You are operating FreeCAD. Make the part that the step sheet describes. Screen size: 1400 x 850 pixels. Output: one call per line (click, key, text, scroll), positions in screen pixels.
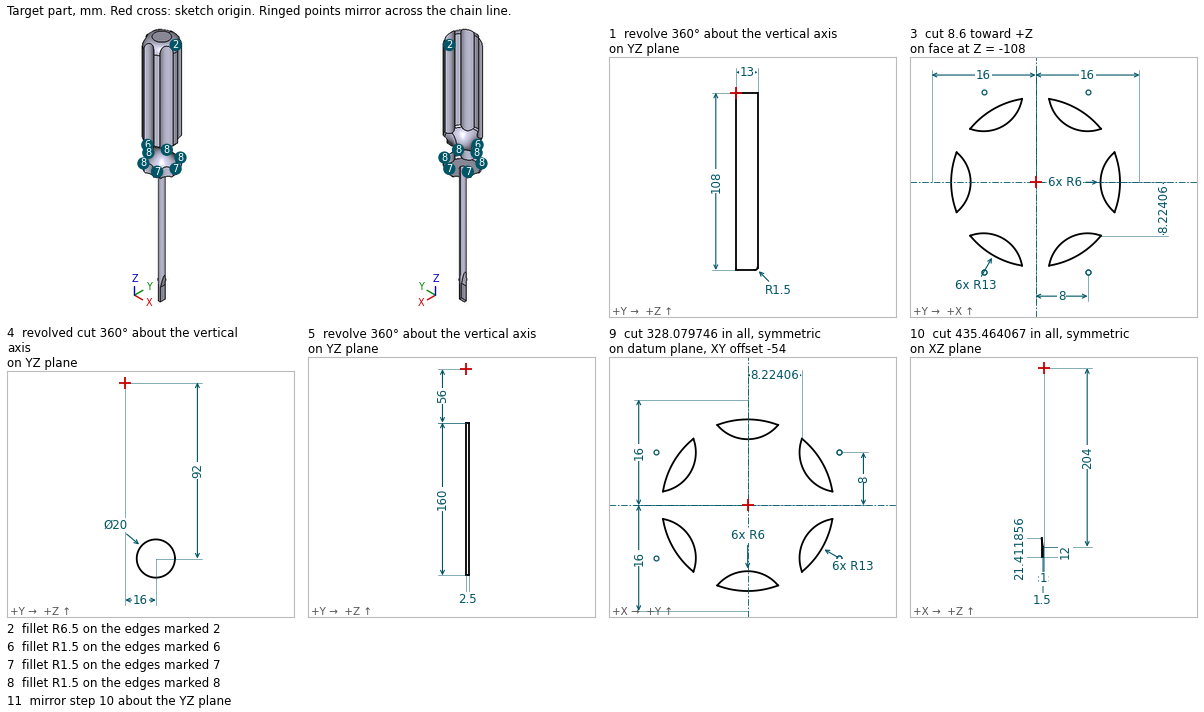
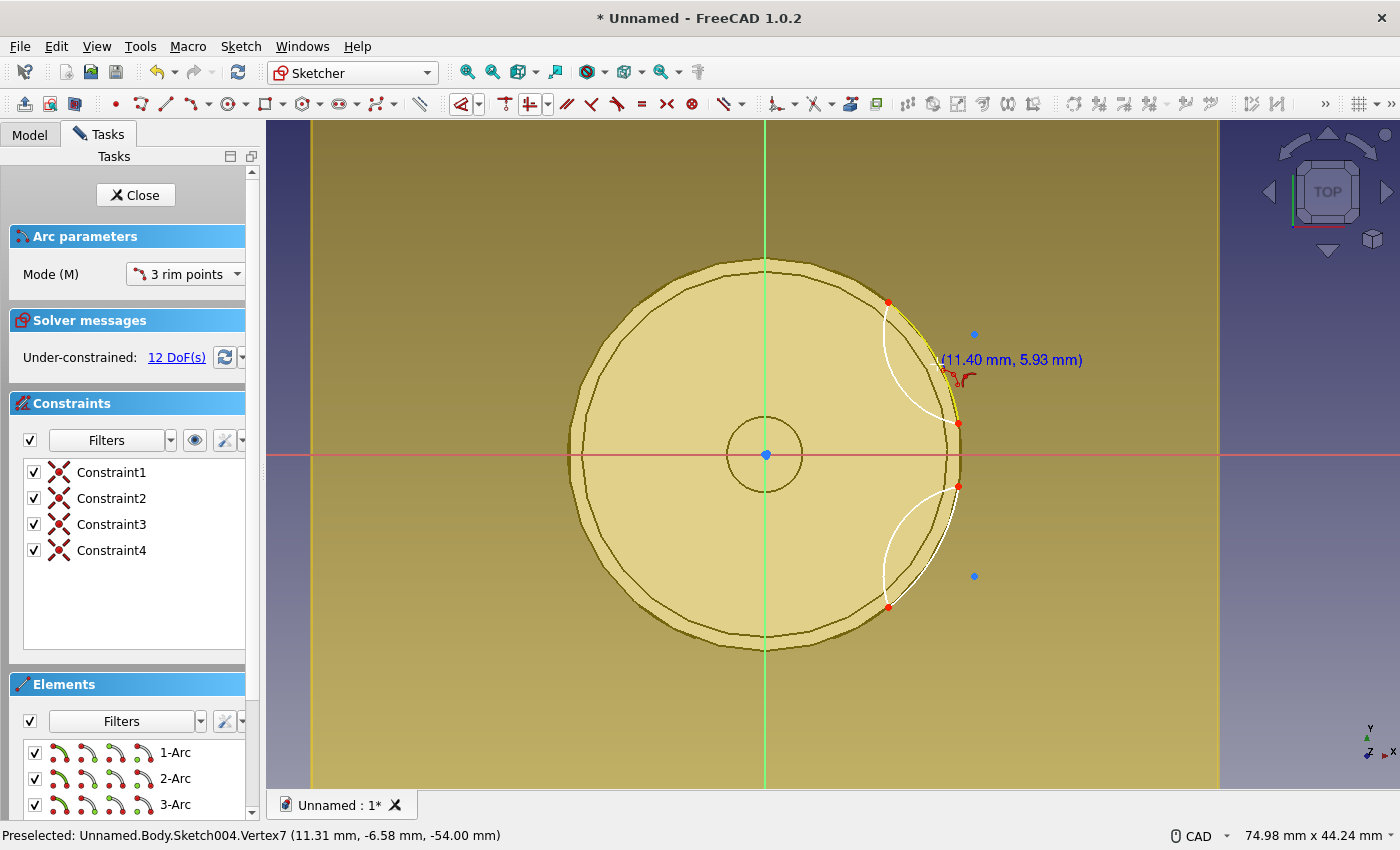
click(834, 638)
click(695, 638)
click(781, 607)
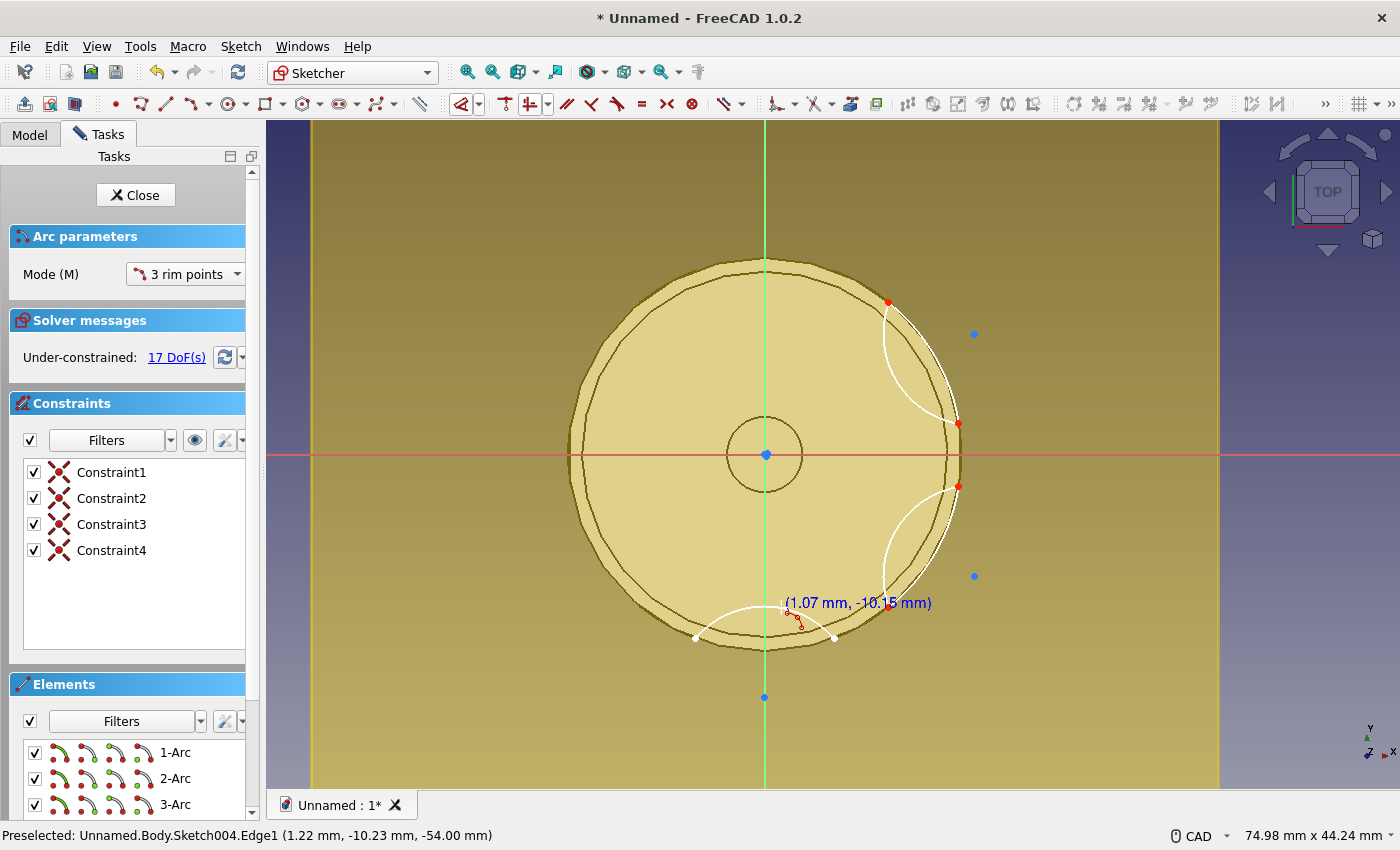
click(695, 639)
click(834, 639)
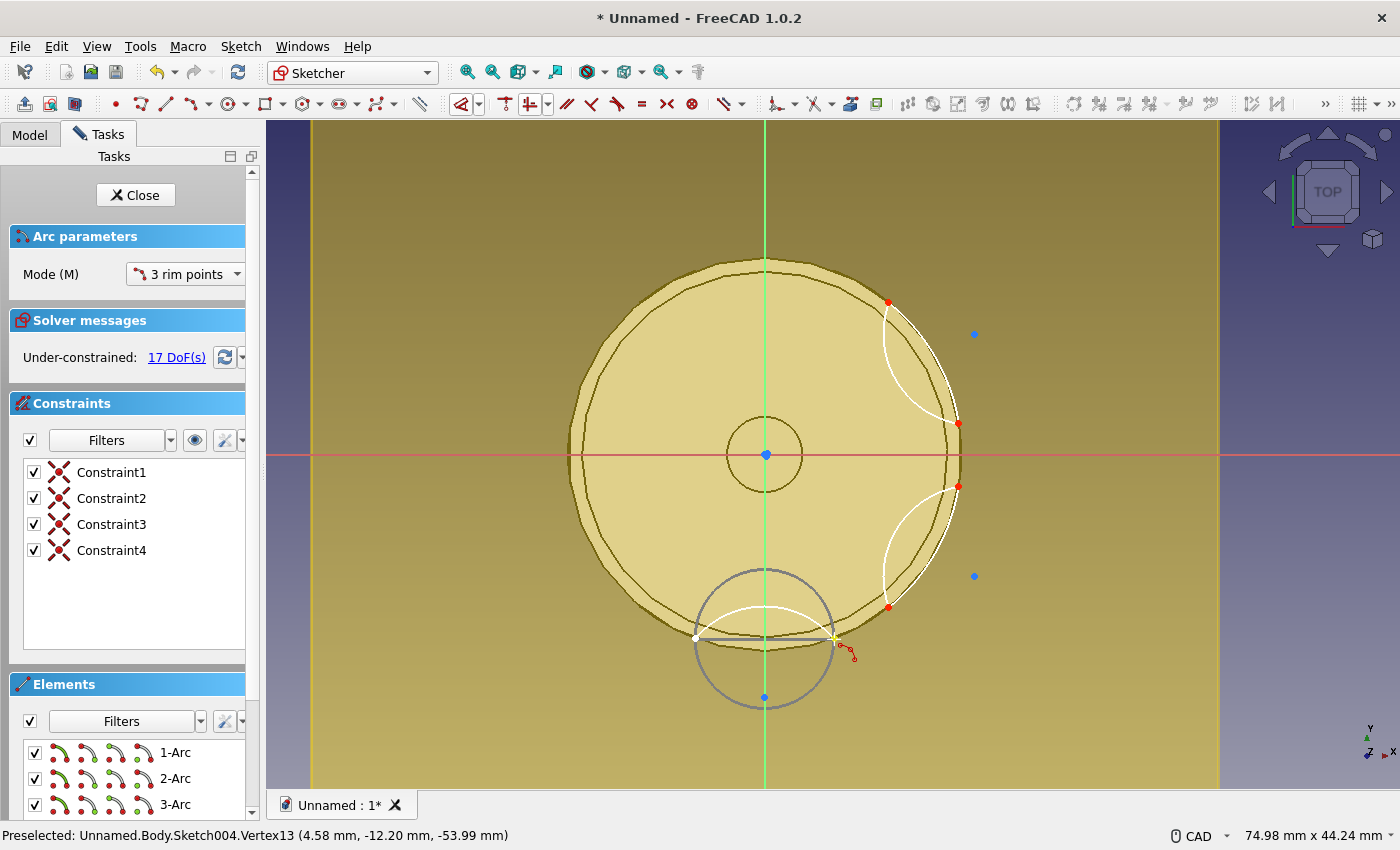
scroll(751, 651, up, 2)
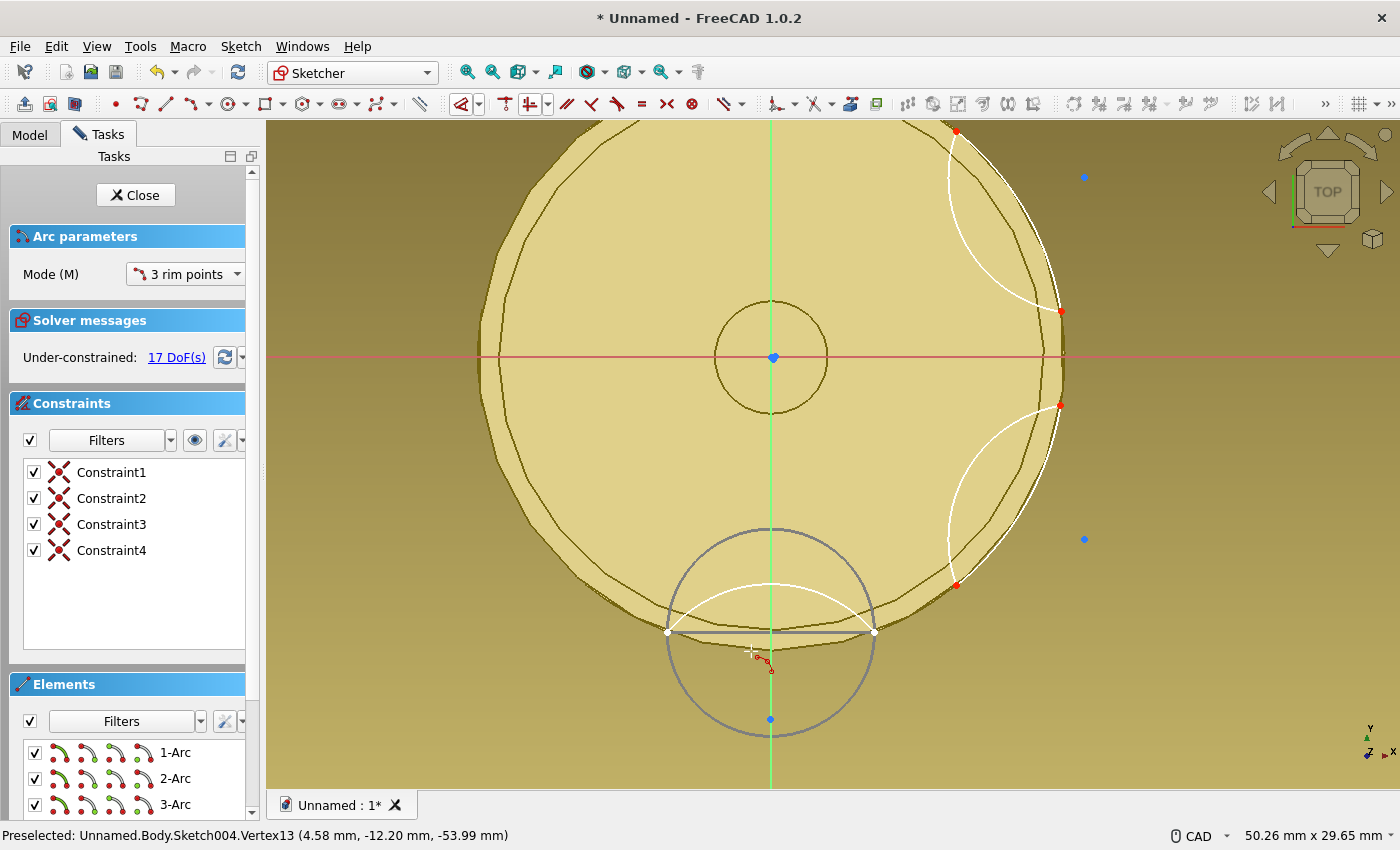
click(750, 650)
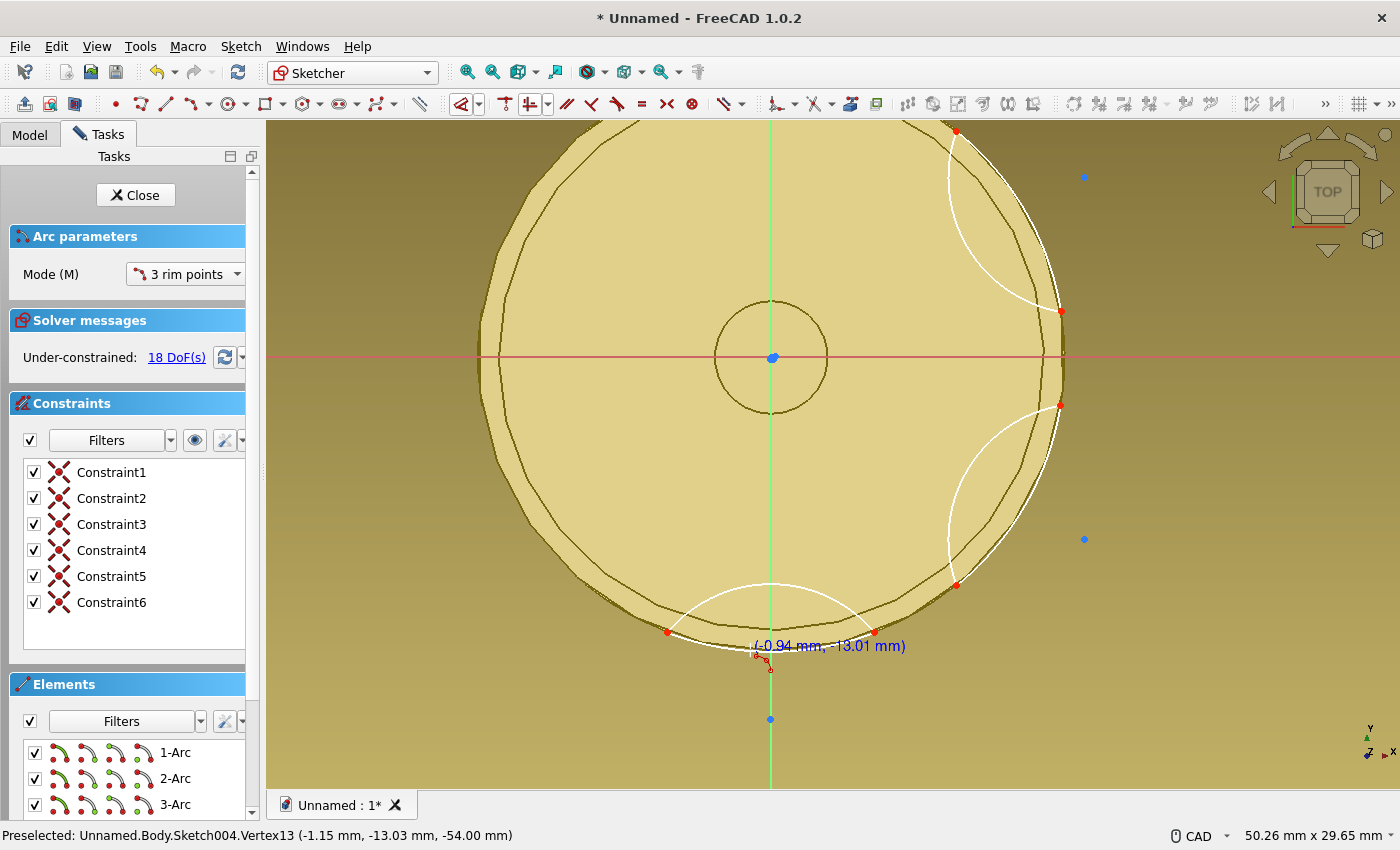
click(482, 405)
click(586, 585)
click(517, 504)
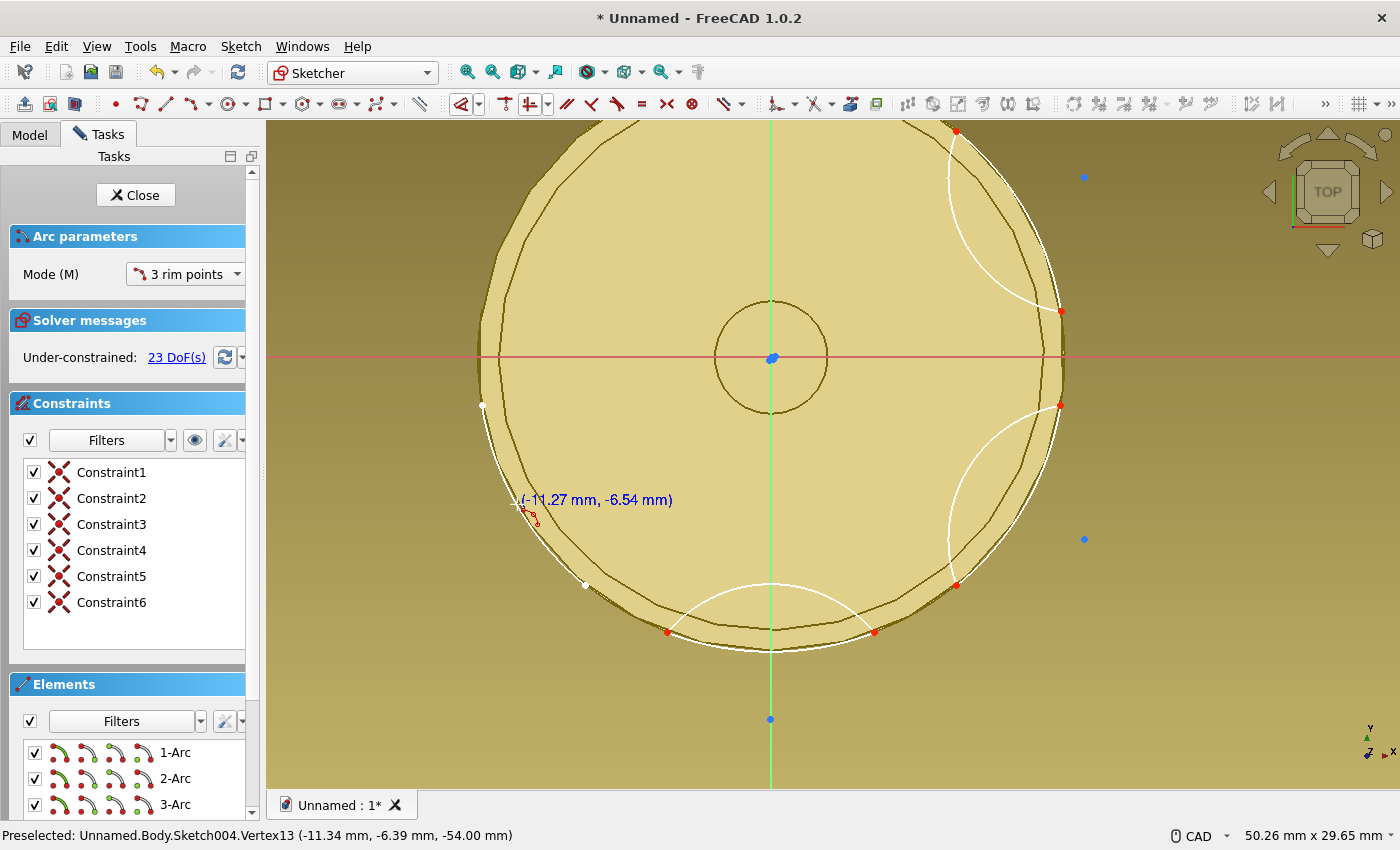
click(586, 586)
click(482, 406)
click(576, 470)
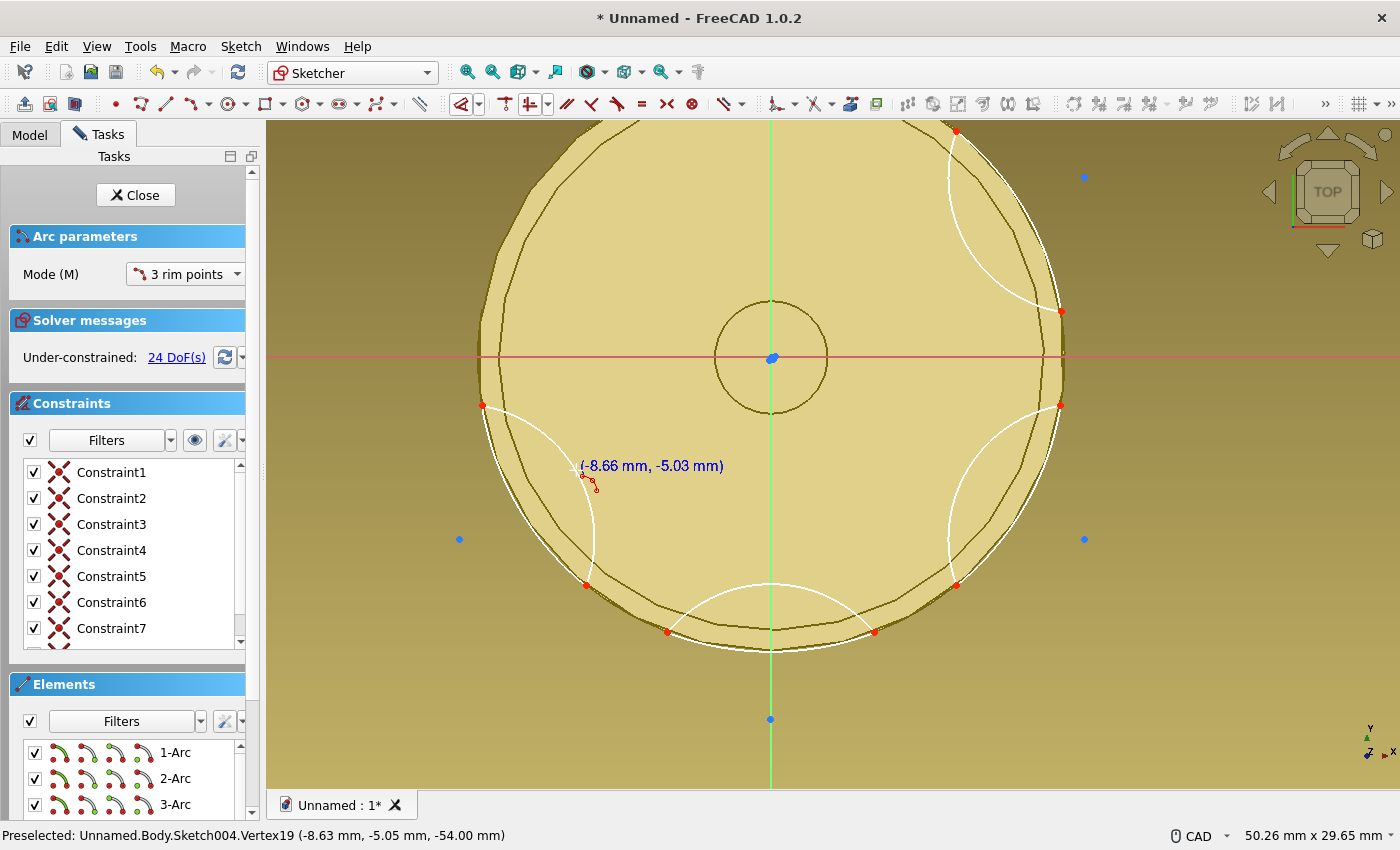
click(482, 310)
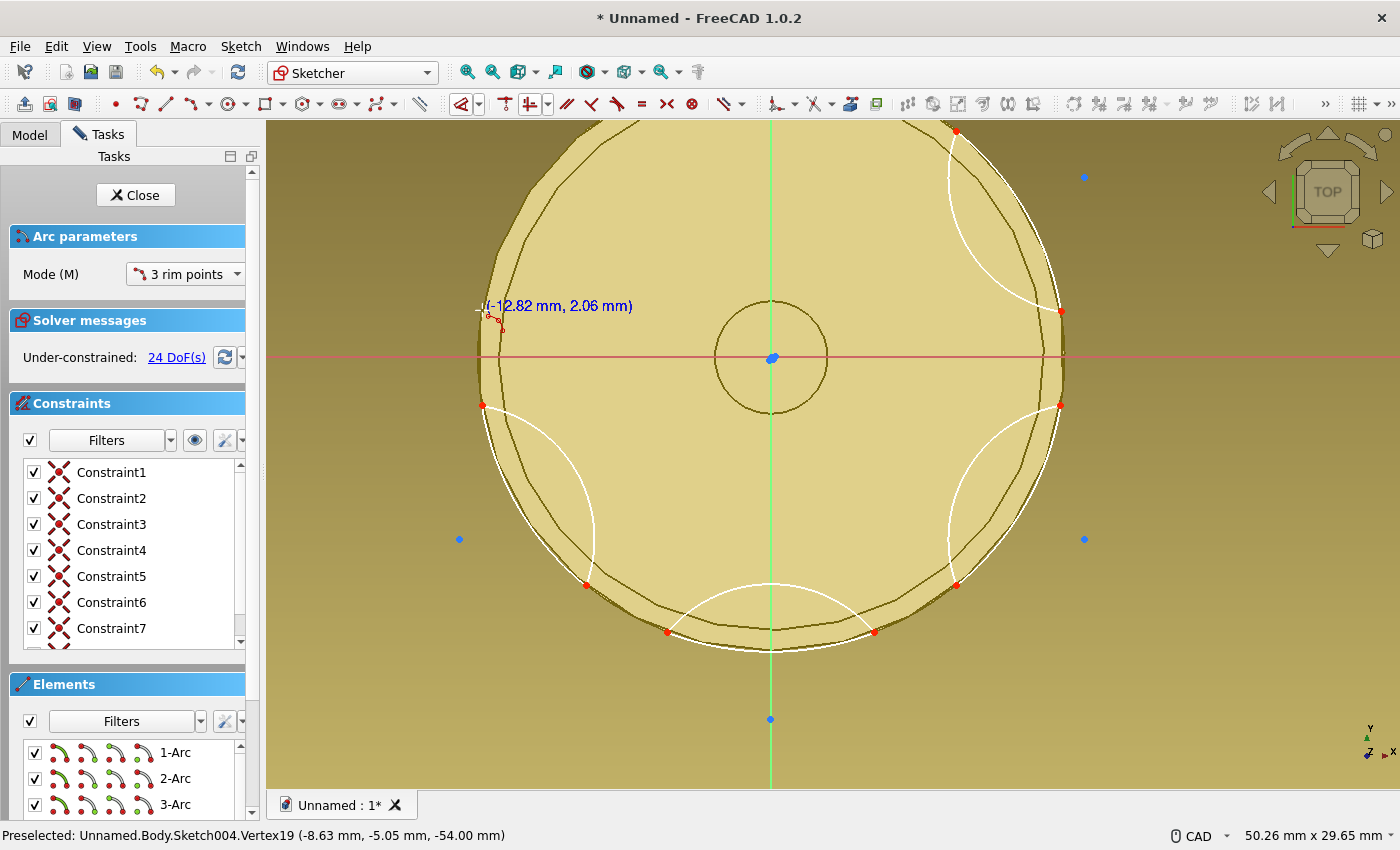
scroll(751, 652, down, 2)